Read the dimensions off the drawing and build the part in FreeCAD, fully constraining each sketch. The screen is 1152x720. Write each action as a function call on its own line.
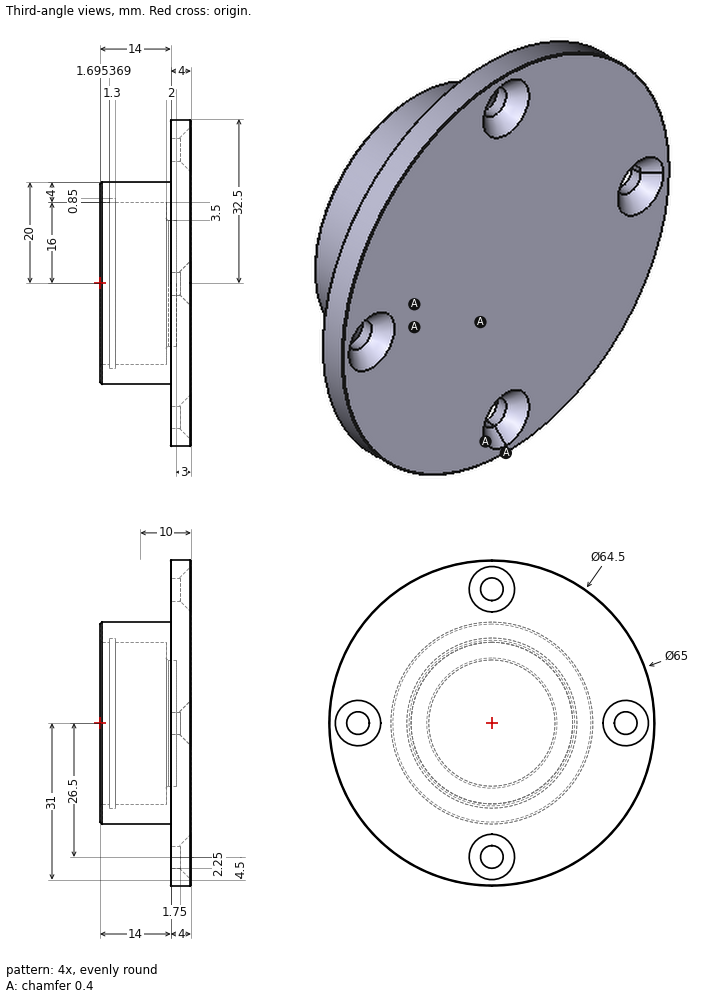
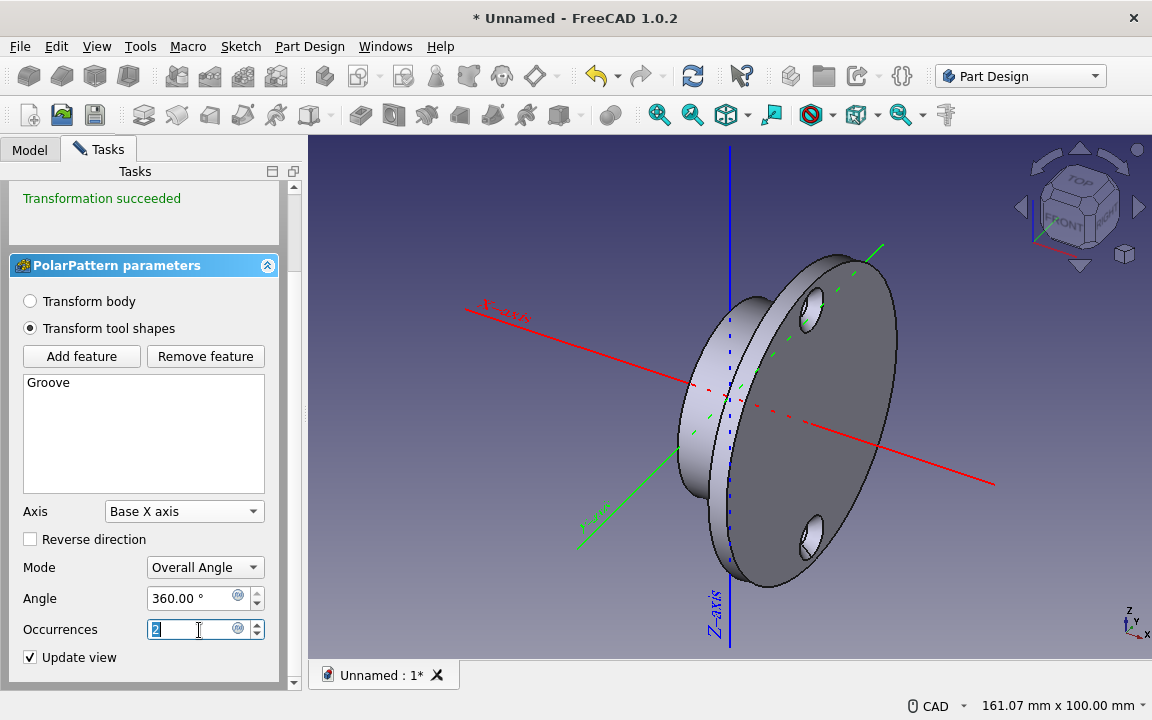
text(4)
key(Tab)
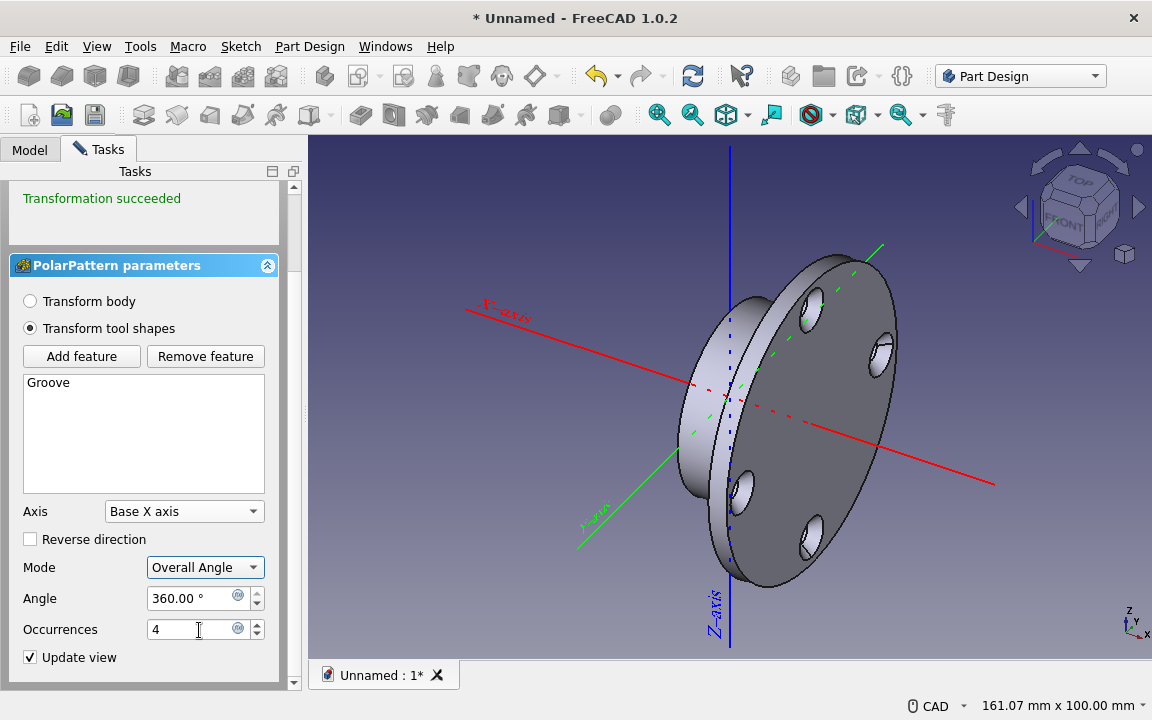
scroll(294, 436, up, 3)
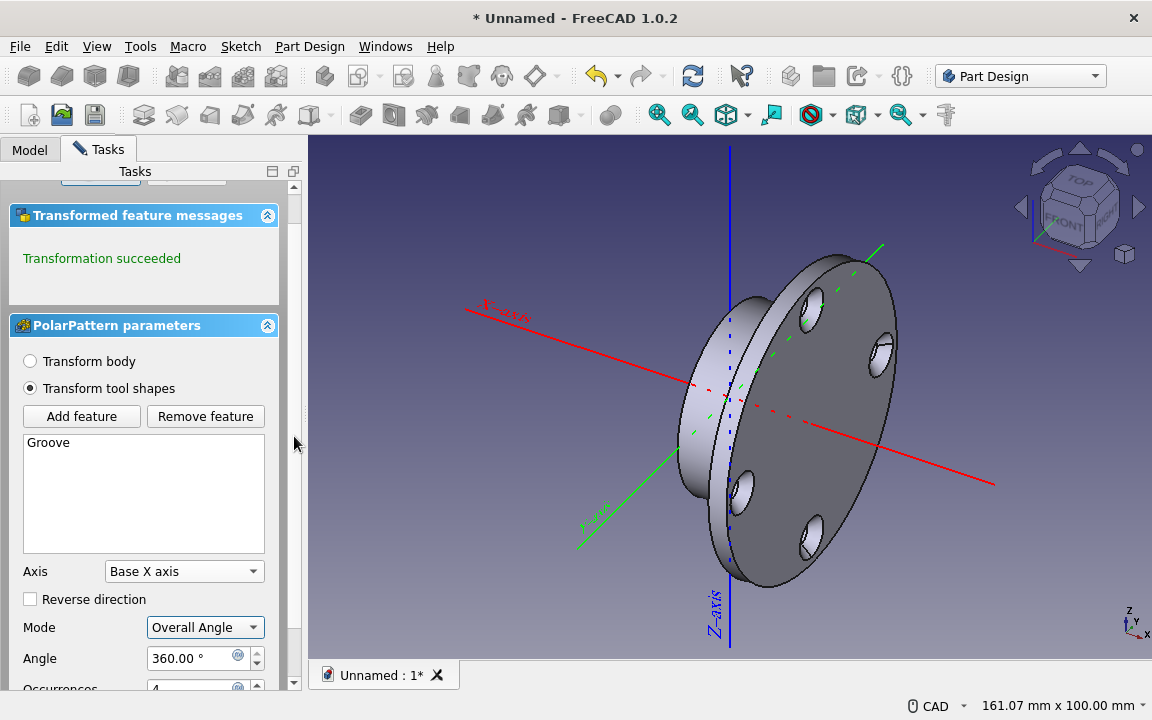
click(101, 210)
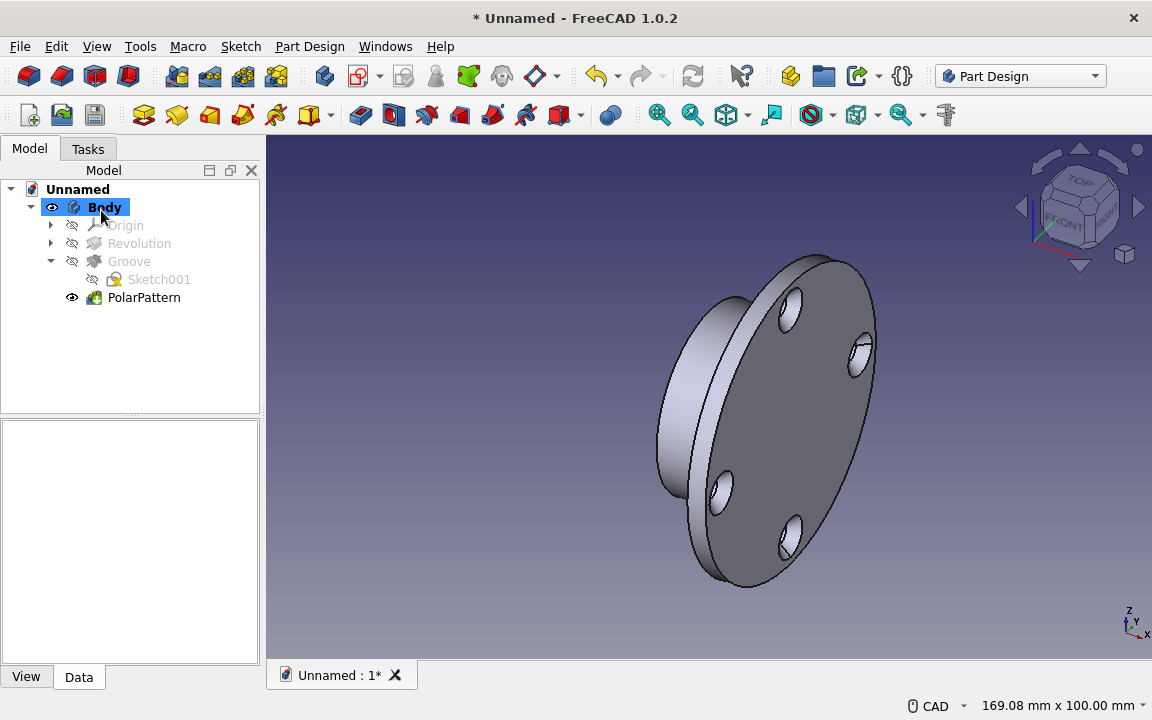
click(706, 508)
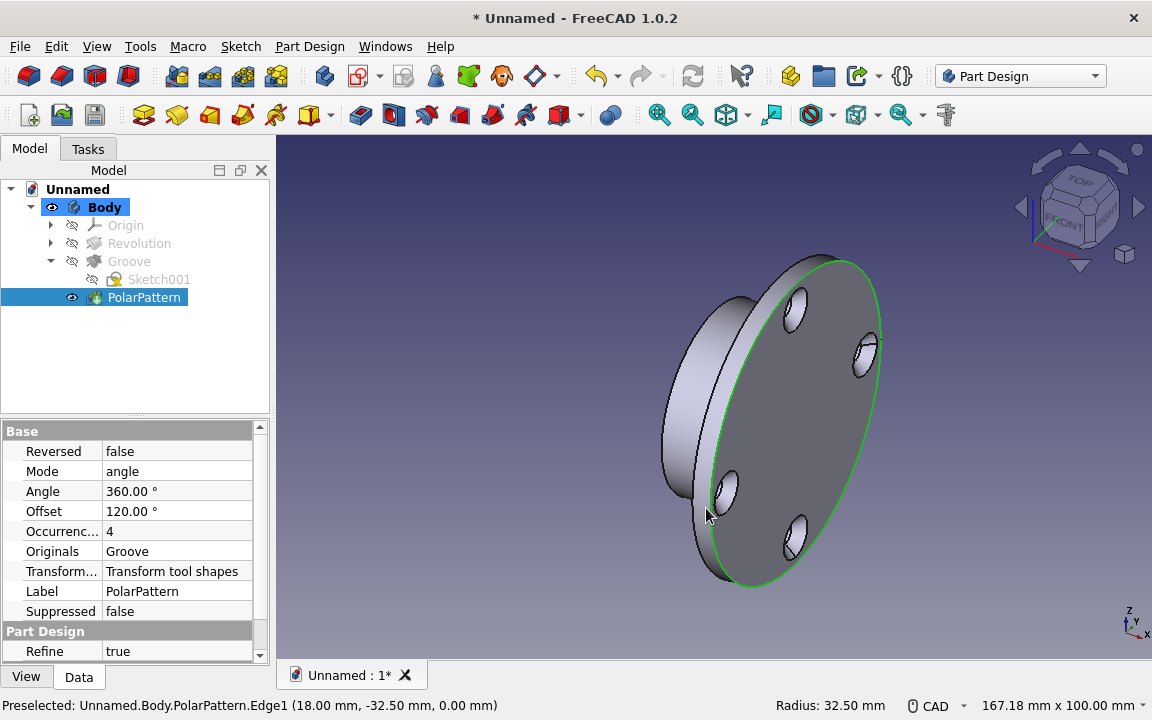
key(0)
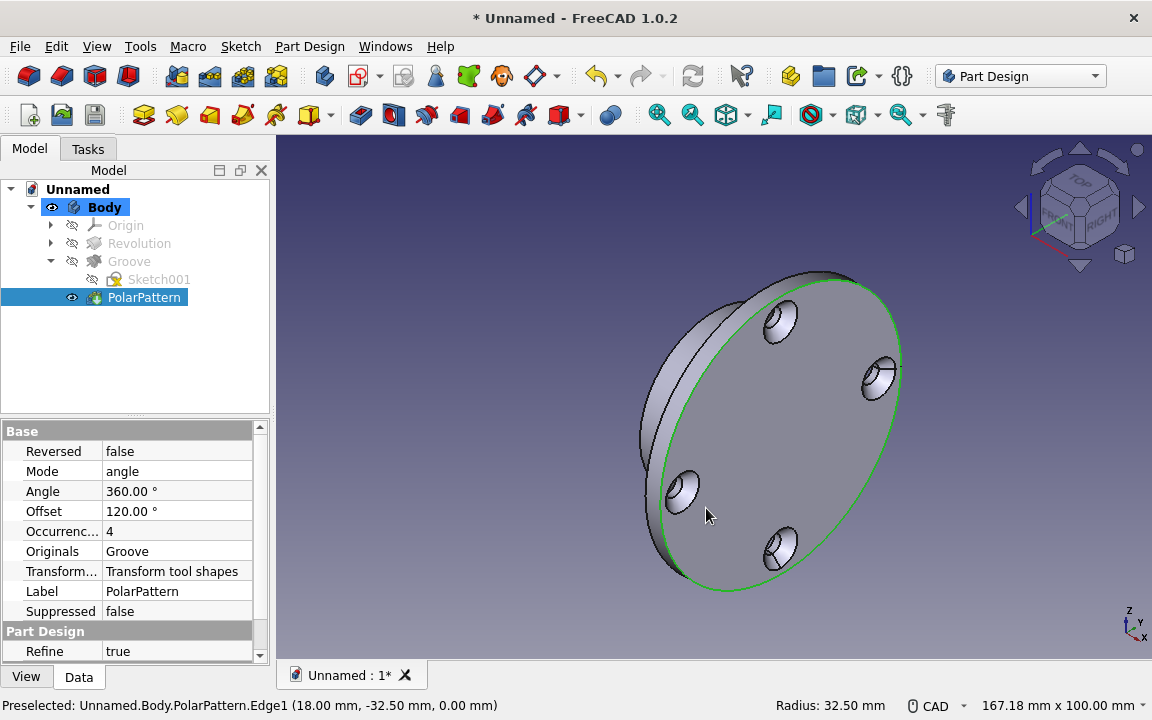
click(668, 400, ctrl)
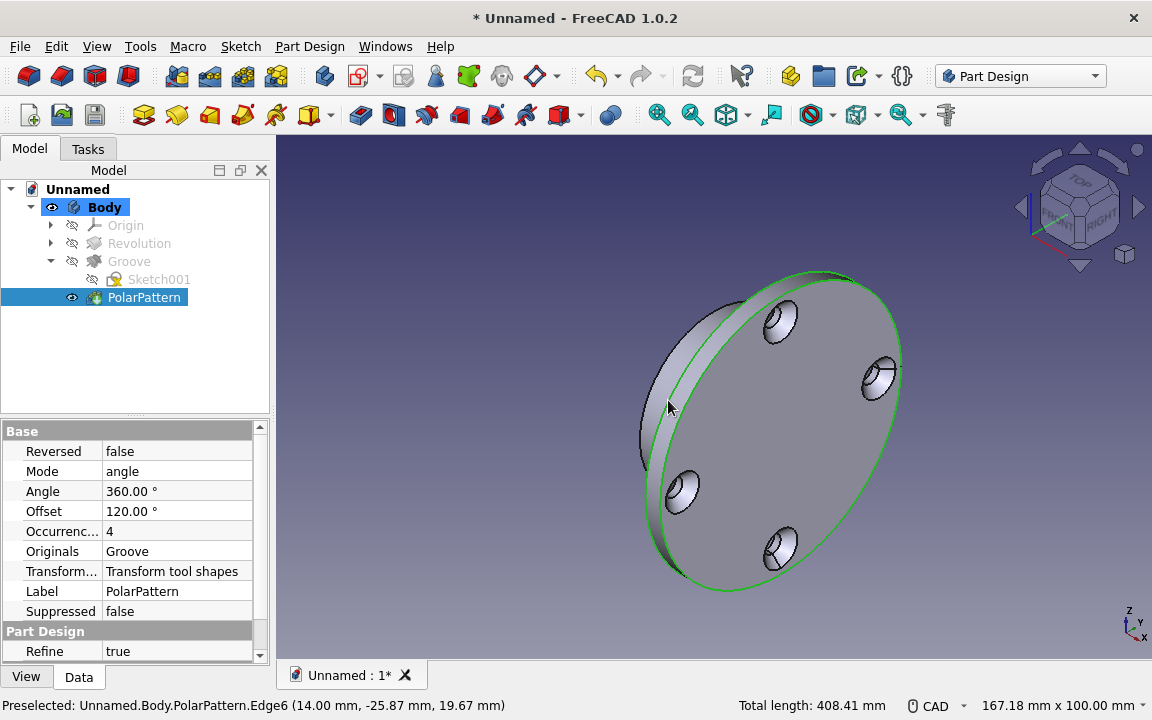
key(2)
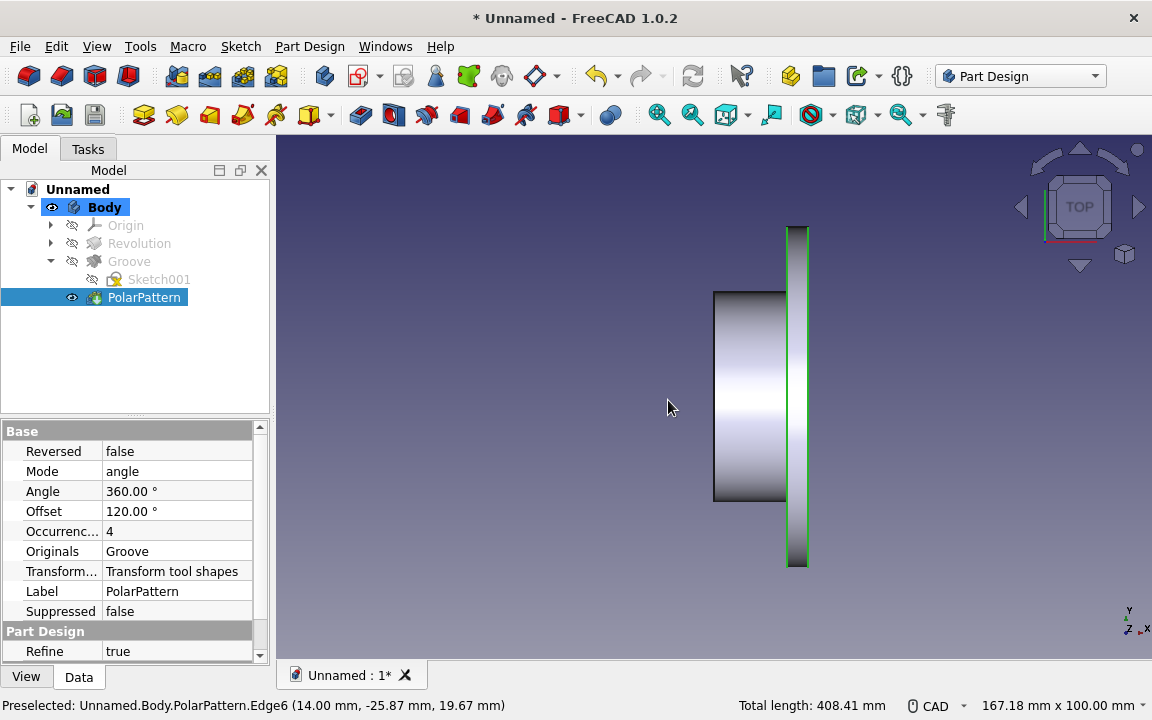
click(714, 481, ctrl)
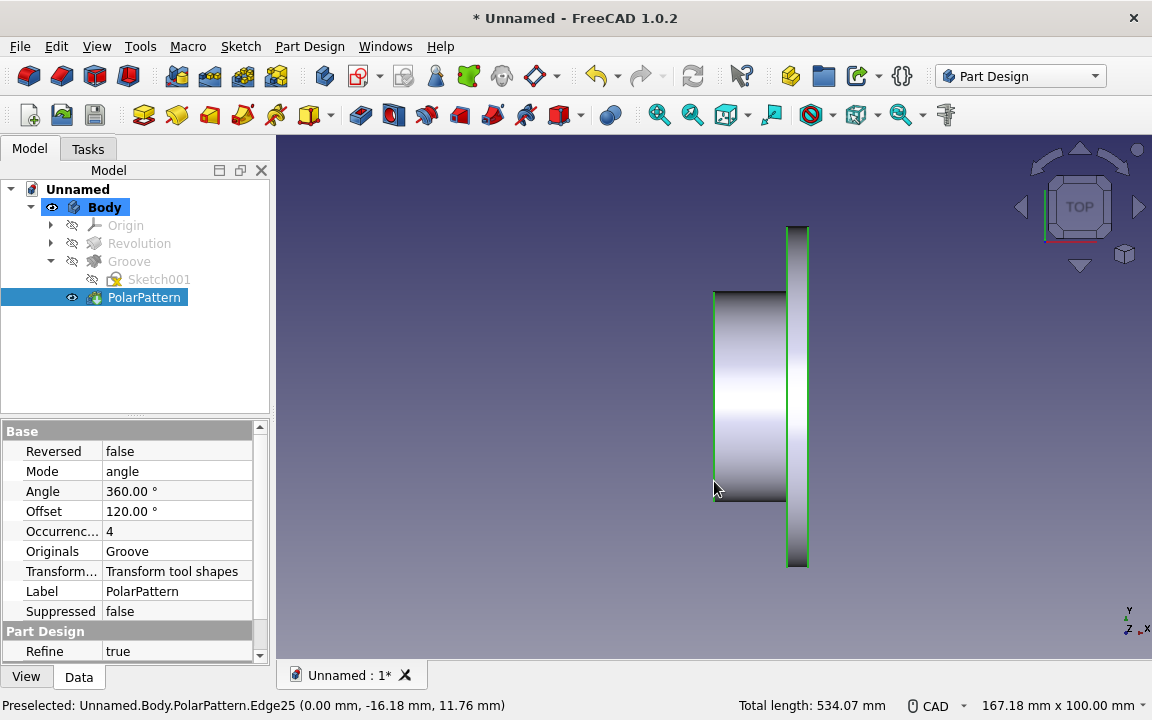
key(1)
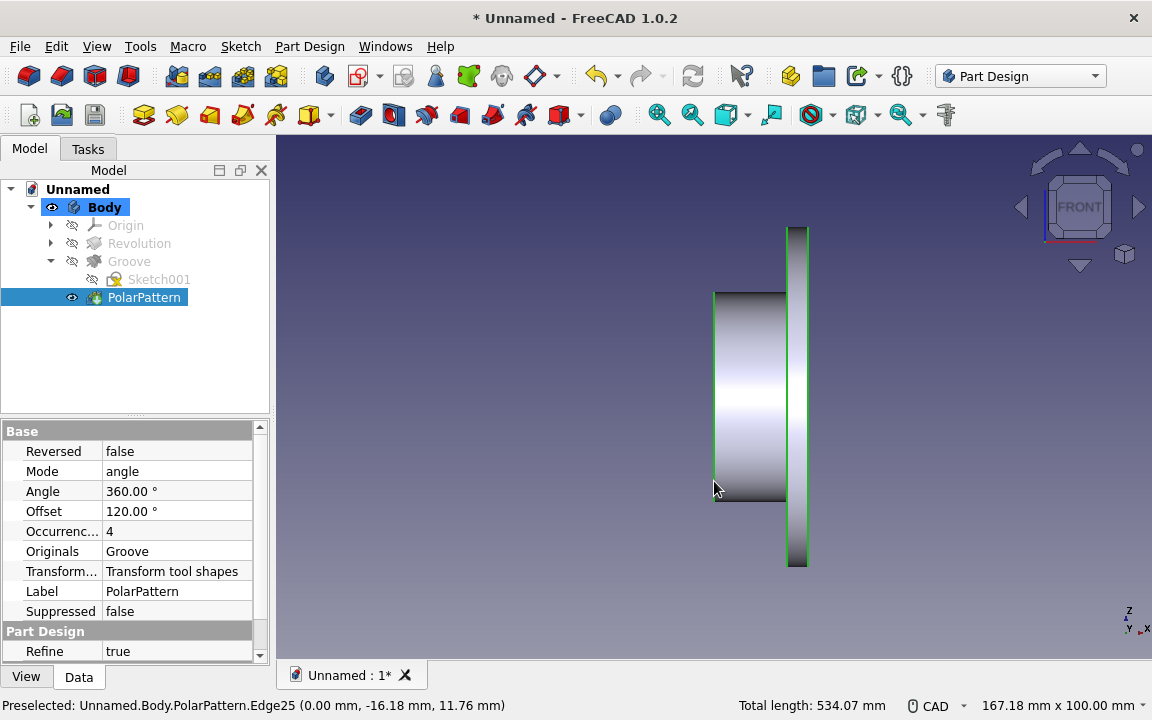
key(3)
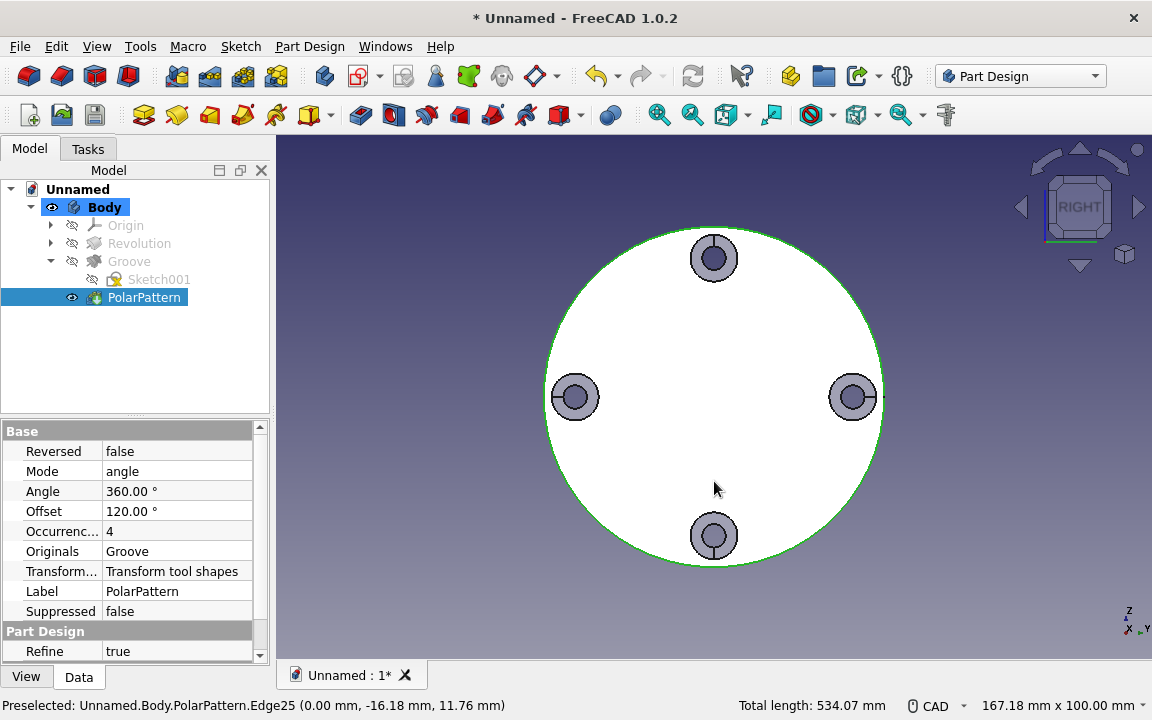
key(5)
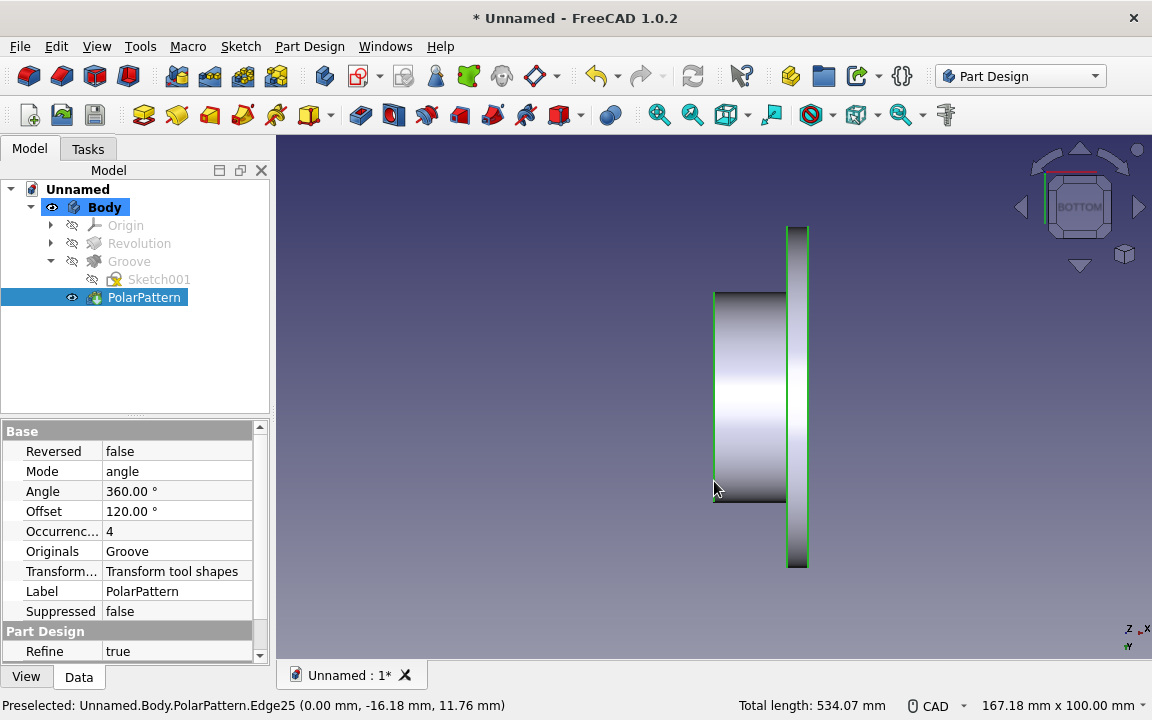
key(4)